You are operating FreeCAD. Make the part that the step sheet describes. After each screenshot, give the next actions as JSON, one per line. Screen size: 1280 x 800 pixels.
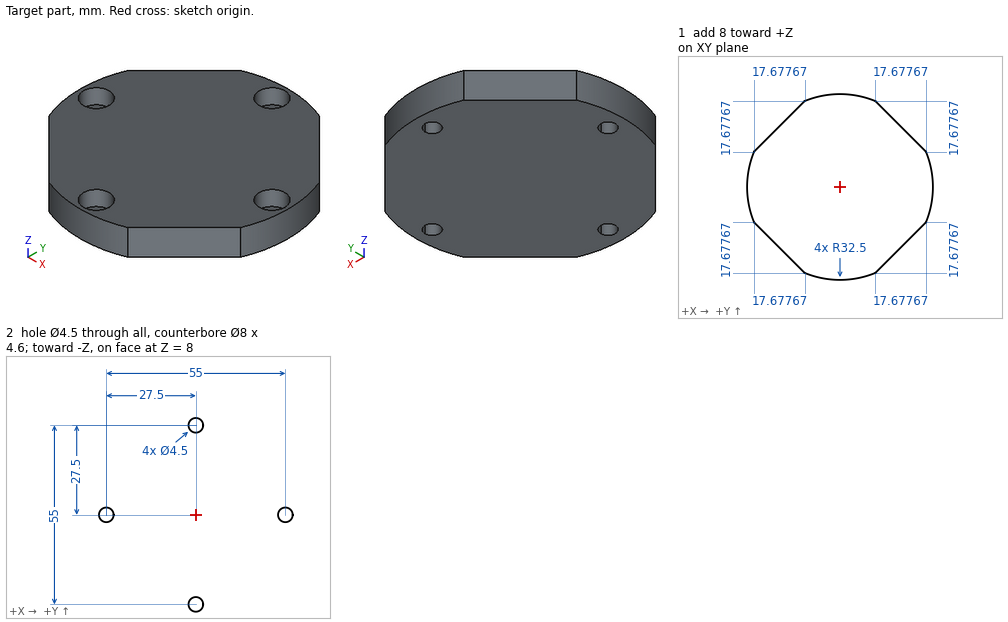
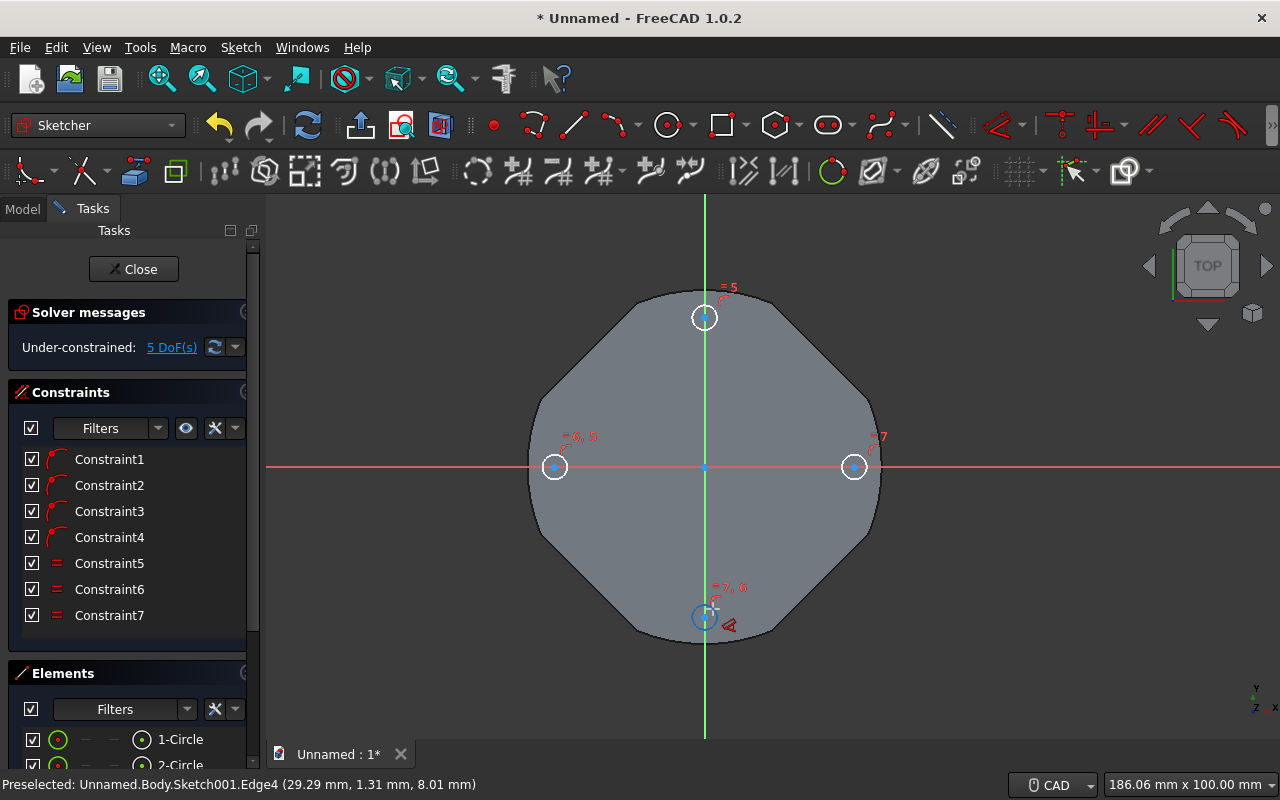
{"action": "scroll", "coordinate": [713, 309], "scroll_direction": "up", "scroll_amount": 3}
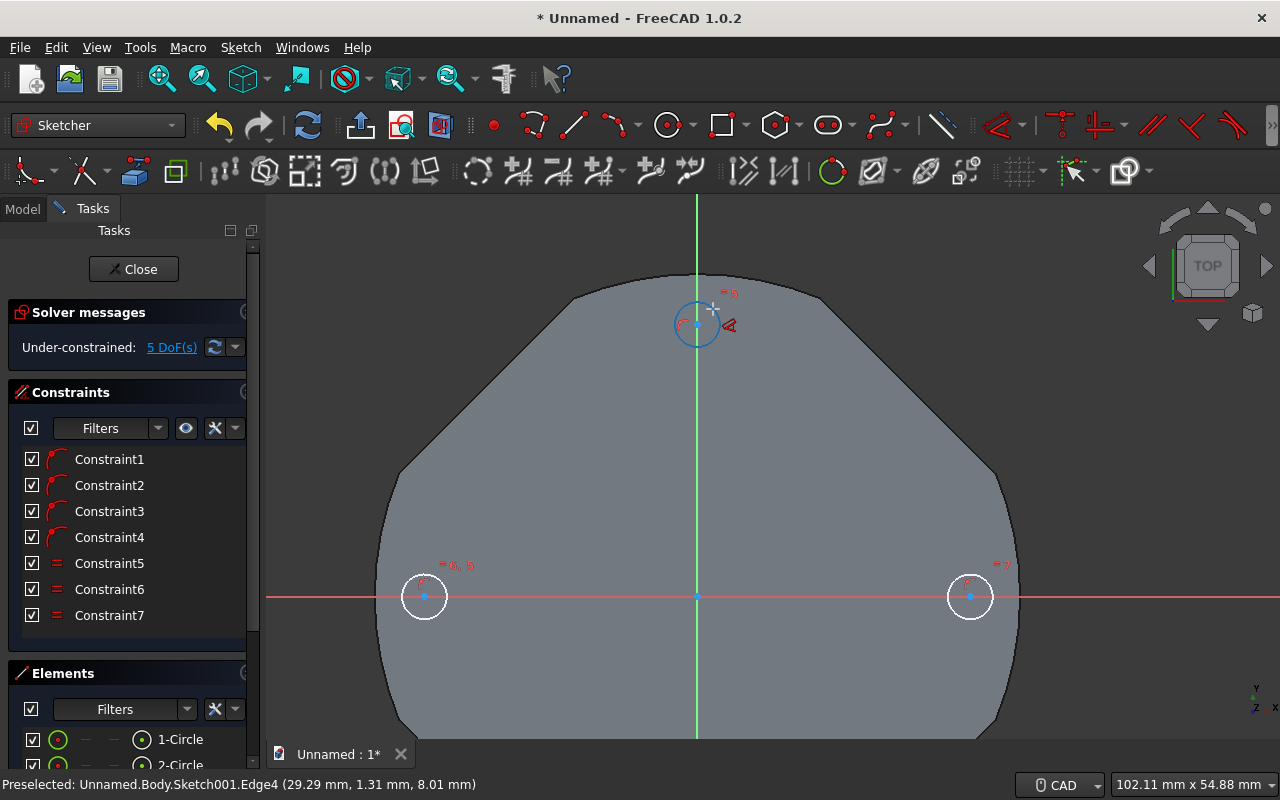
{"action": "left_click", "coordinate": [713, 309]}
{"action": "left_click", "coordinate": [736, 286]}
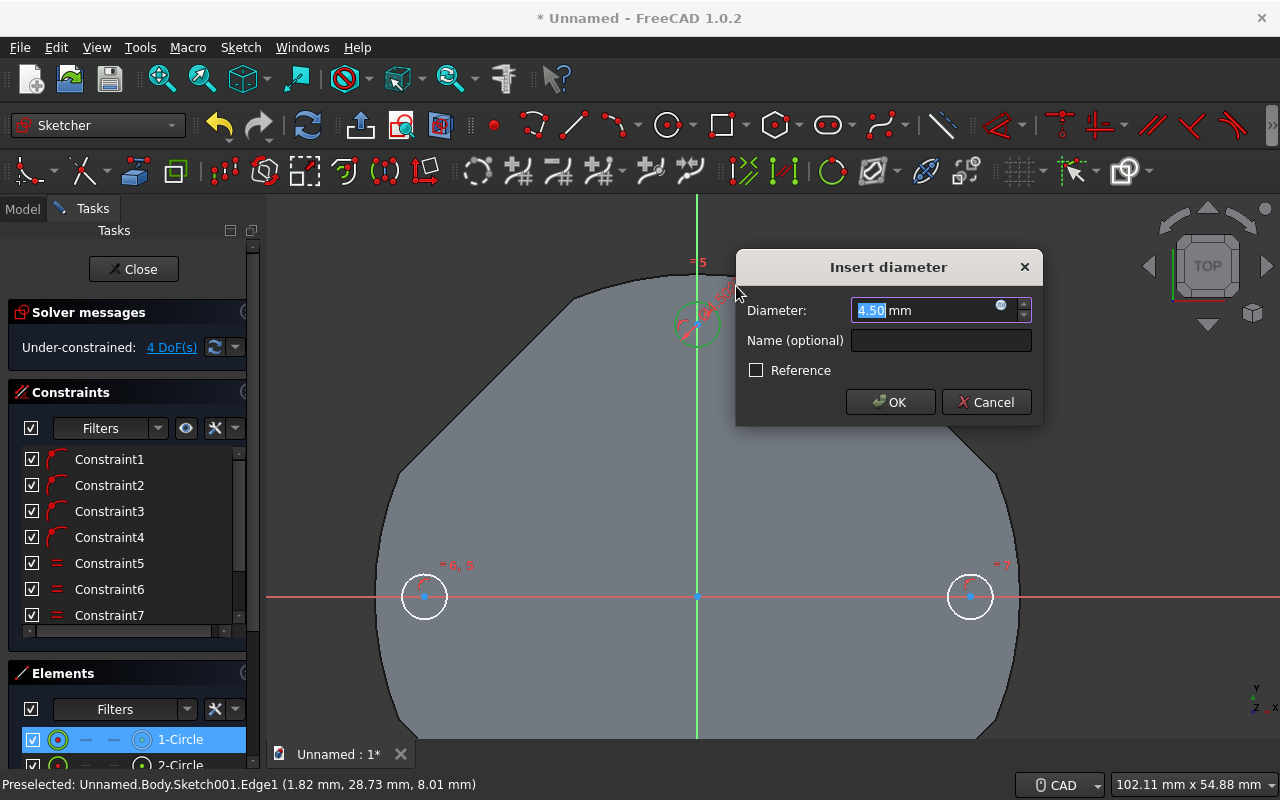
{"action": "type", "text": "4.5"}
{"action": "key", "text": "Return"}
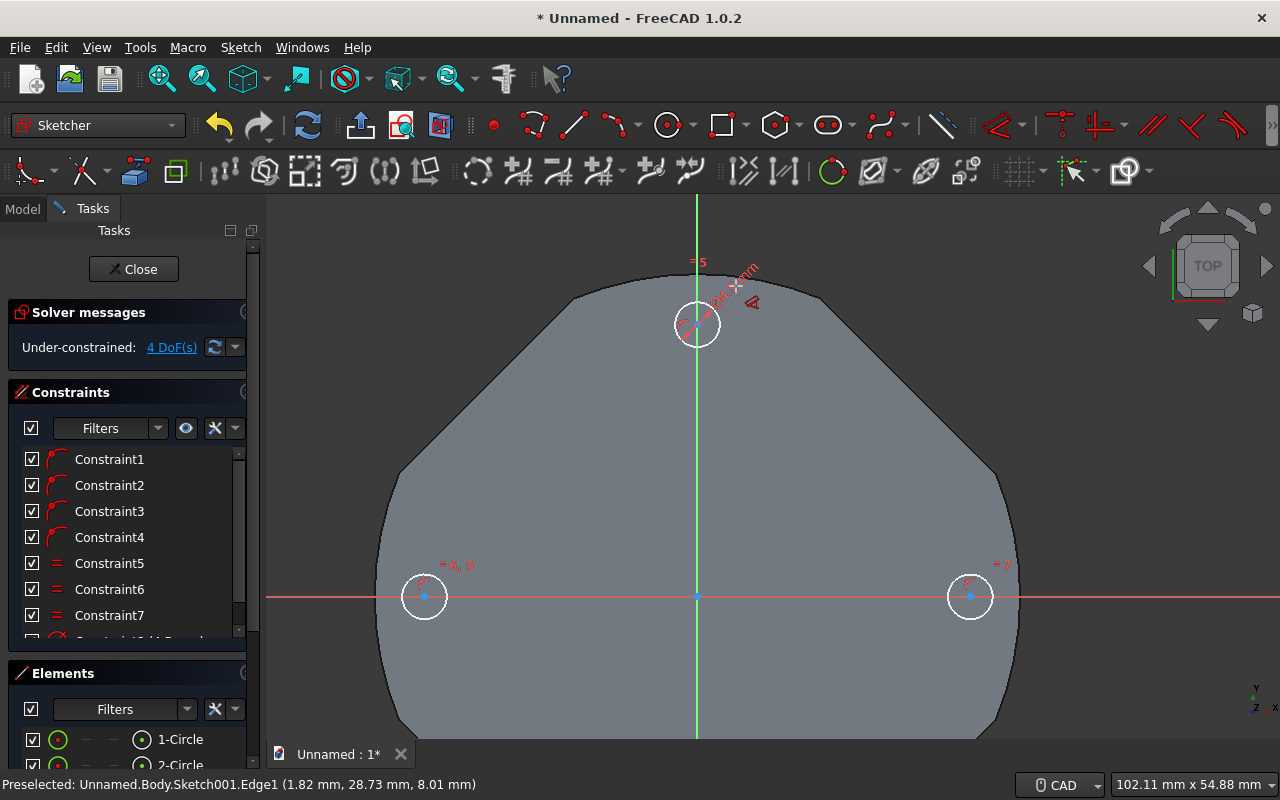
{"action": "left_click", "coordinate": [697, 325]}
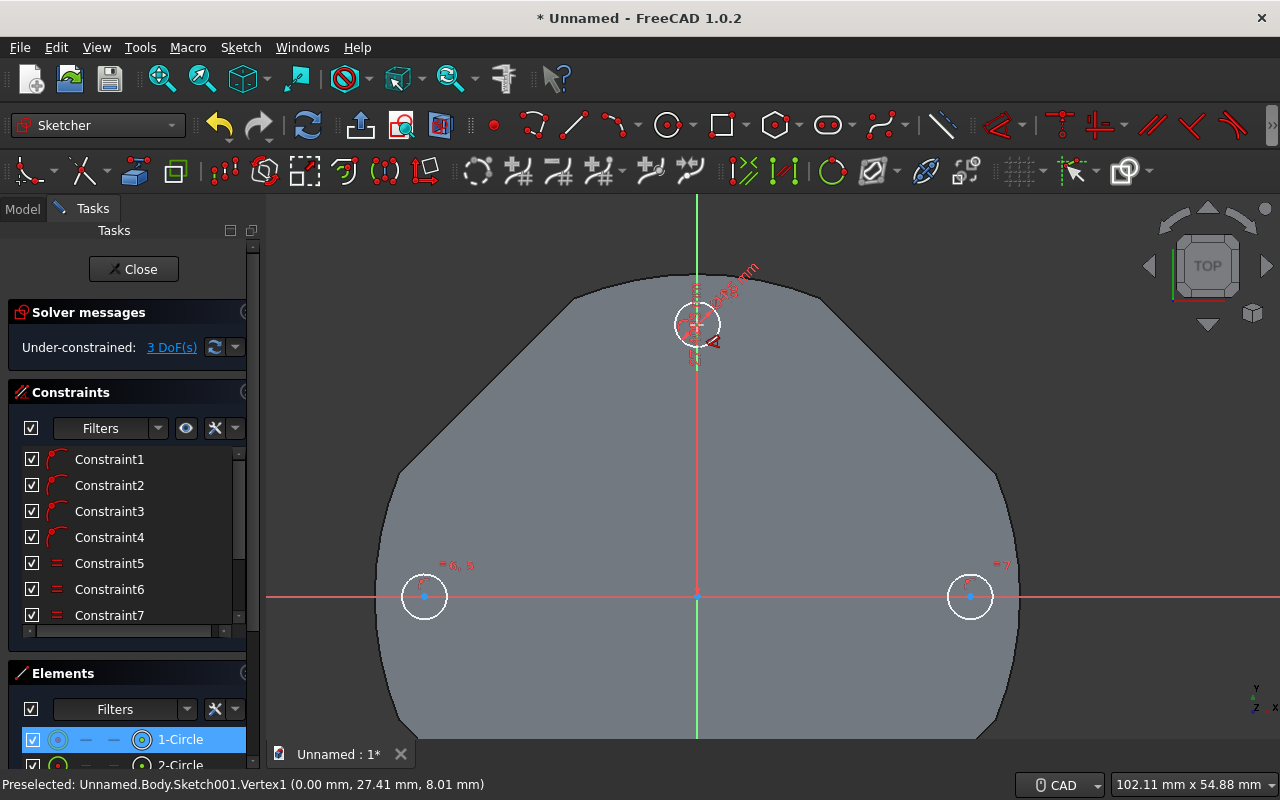
{"action": "scroll", "coordinate": [713, 308], "scroll_direction": "down", "scroll_amount": 3}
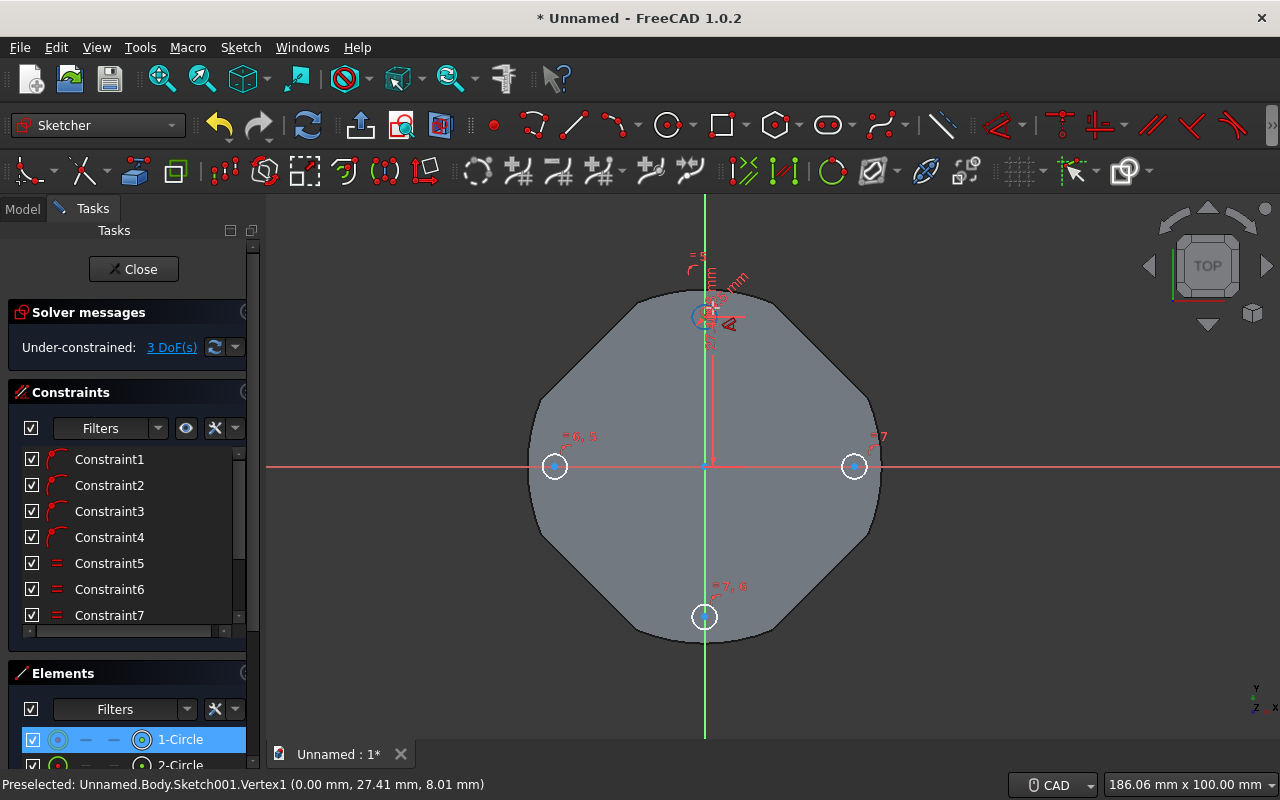
{"action": "left_click", "coordinate": [705, 617]}
{"action": "left_click", "coordinate": [739, 398]}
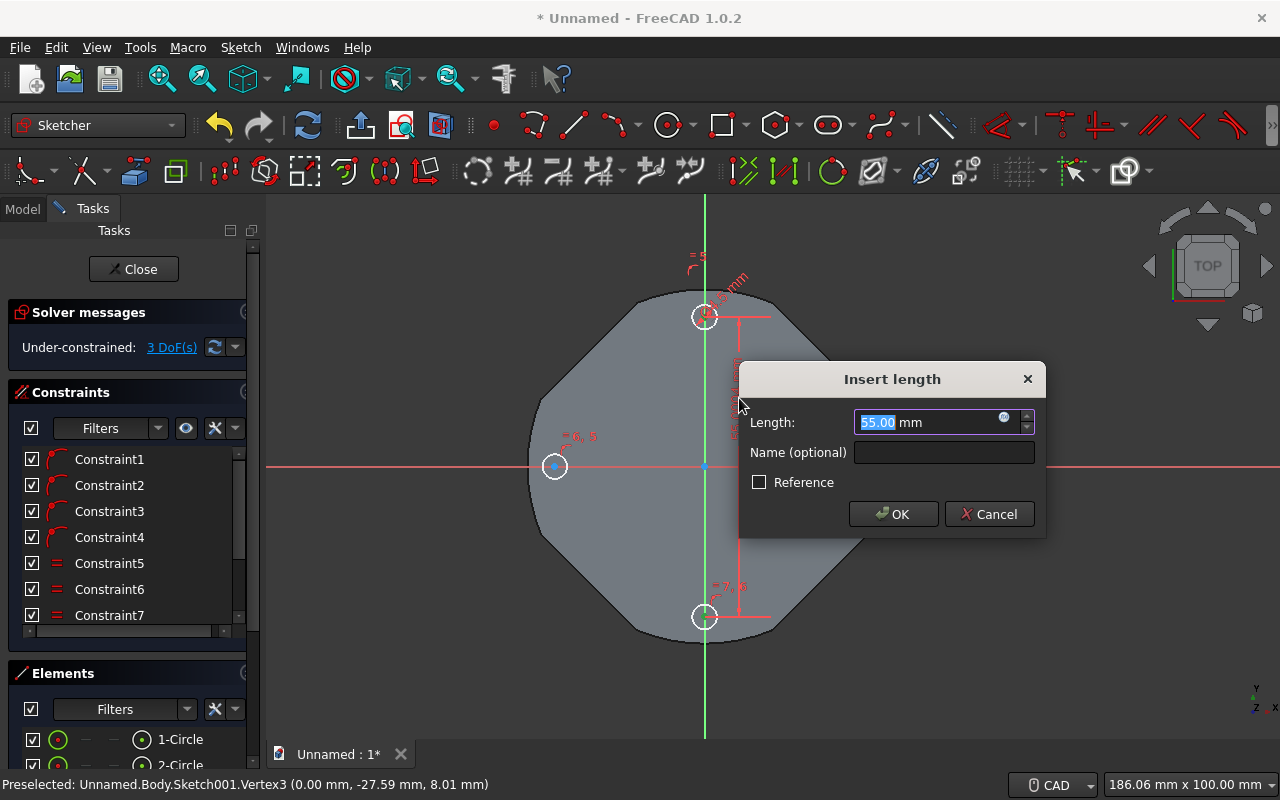
{"action": "type", "text": "55"}
{"action": "key", "text": "Return"}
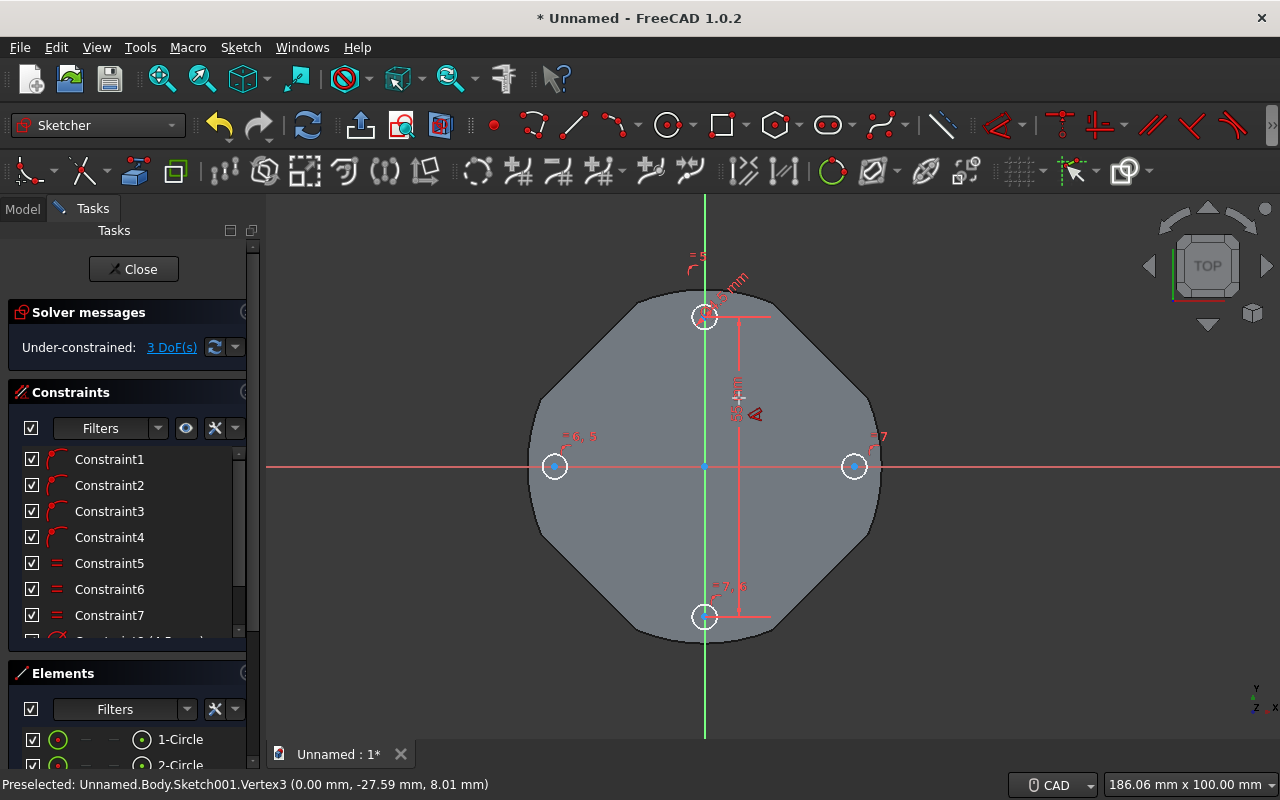
{"action": "left_click", "coordinate": [555, 467]}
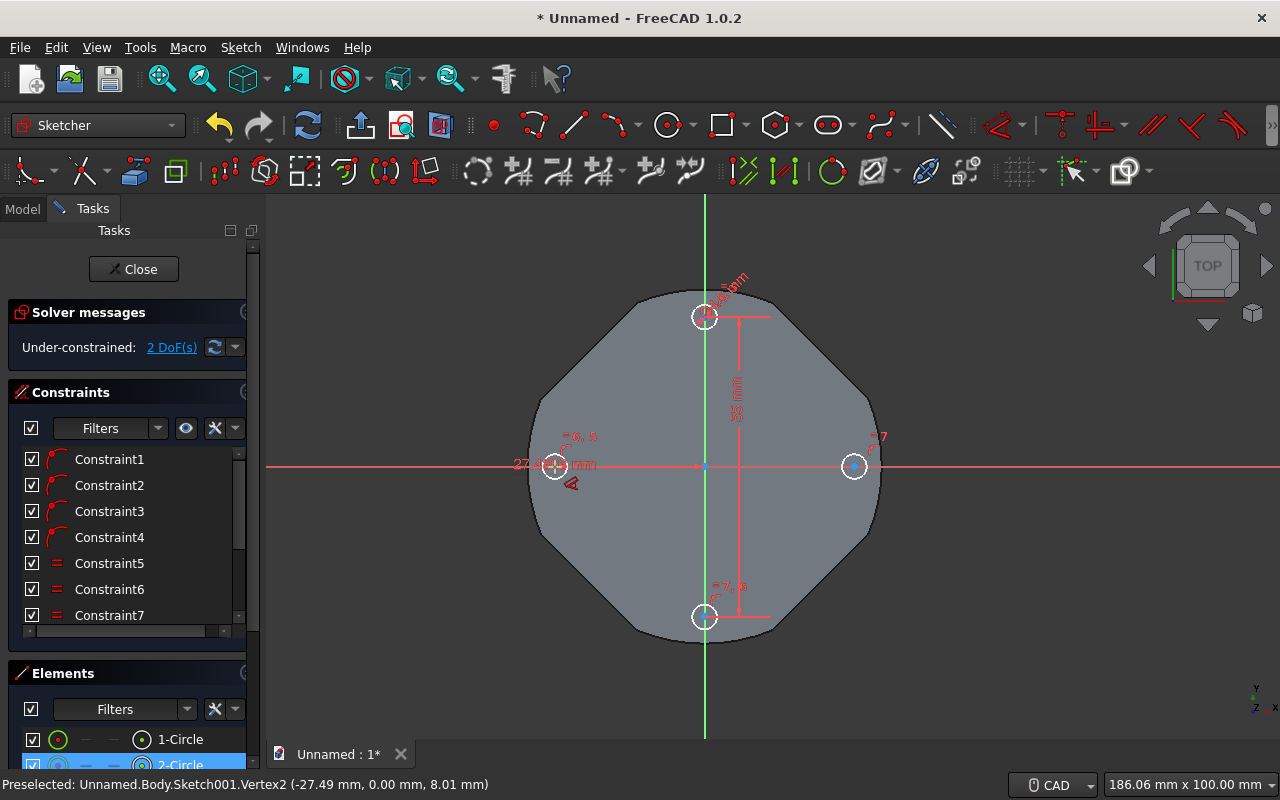
{"action": "left_click", "coordinate": [854, 467]}
{"action": "left_click", "coordinate": [636, 501]}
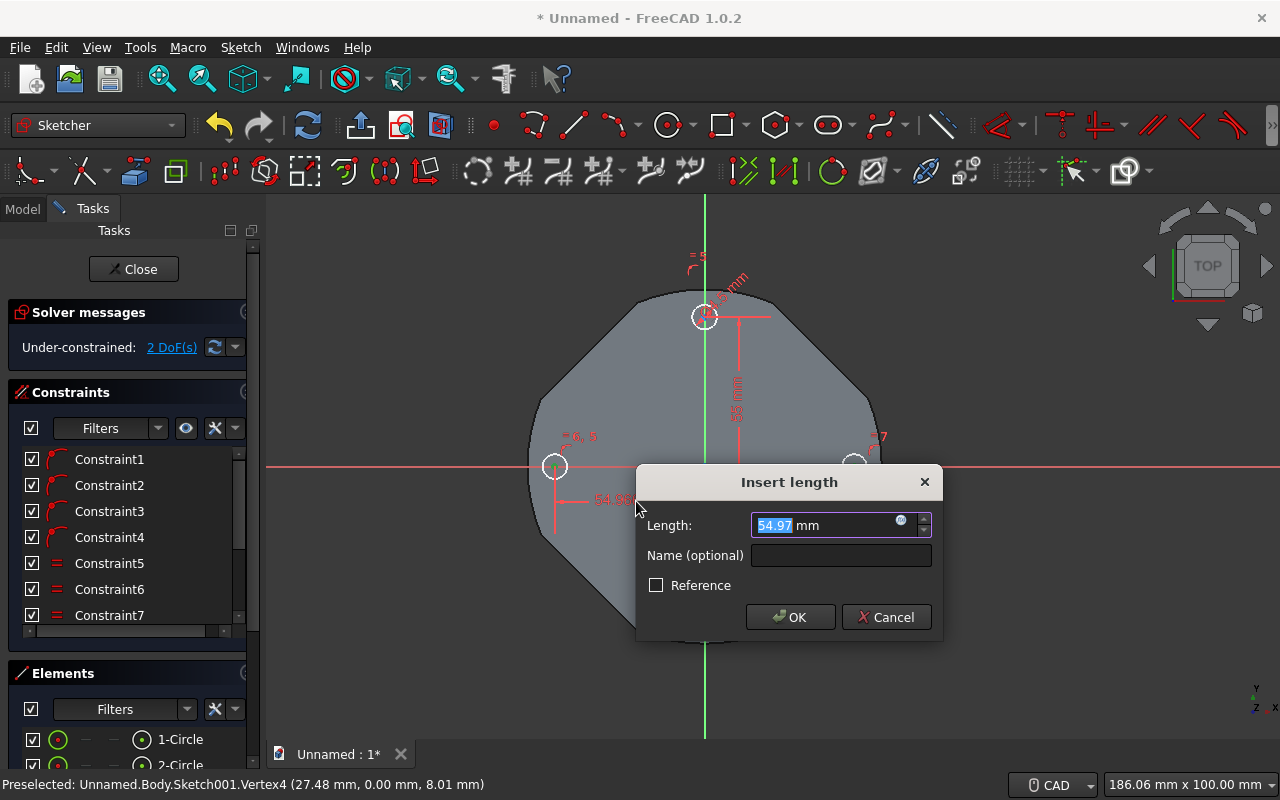
{"action": "type", "text": "55"}
{"action": "key", "text": "Return"}